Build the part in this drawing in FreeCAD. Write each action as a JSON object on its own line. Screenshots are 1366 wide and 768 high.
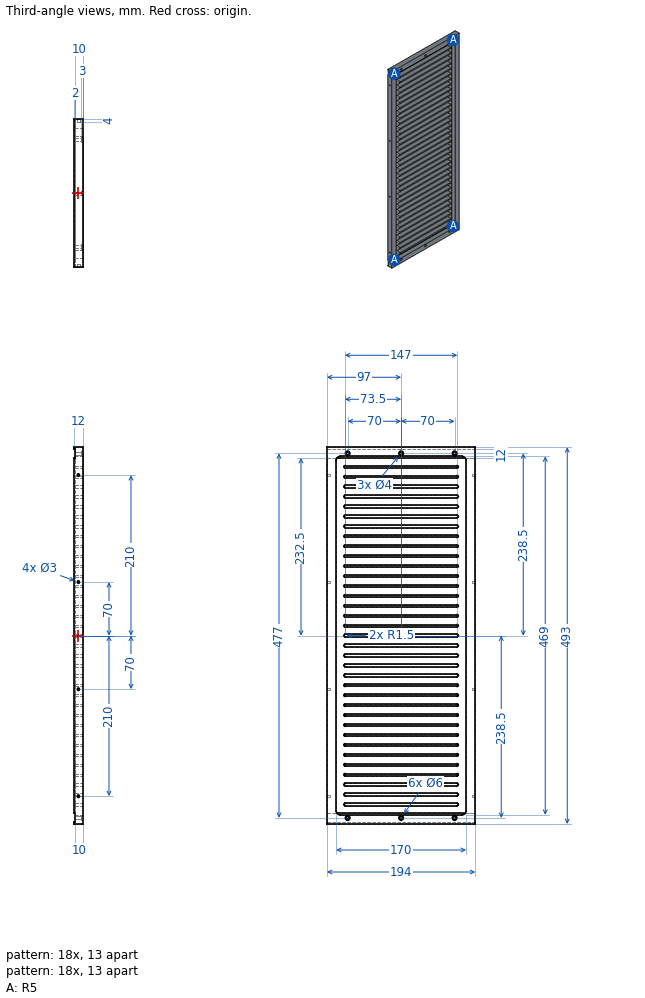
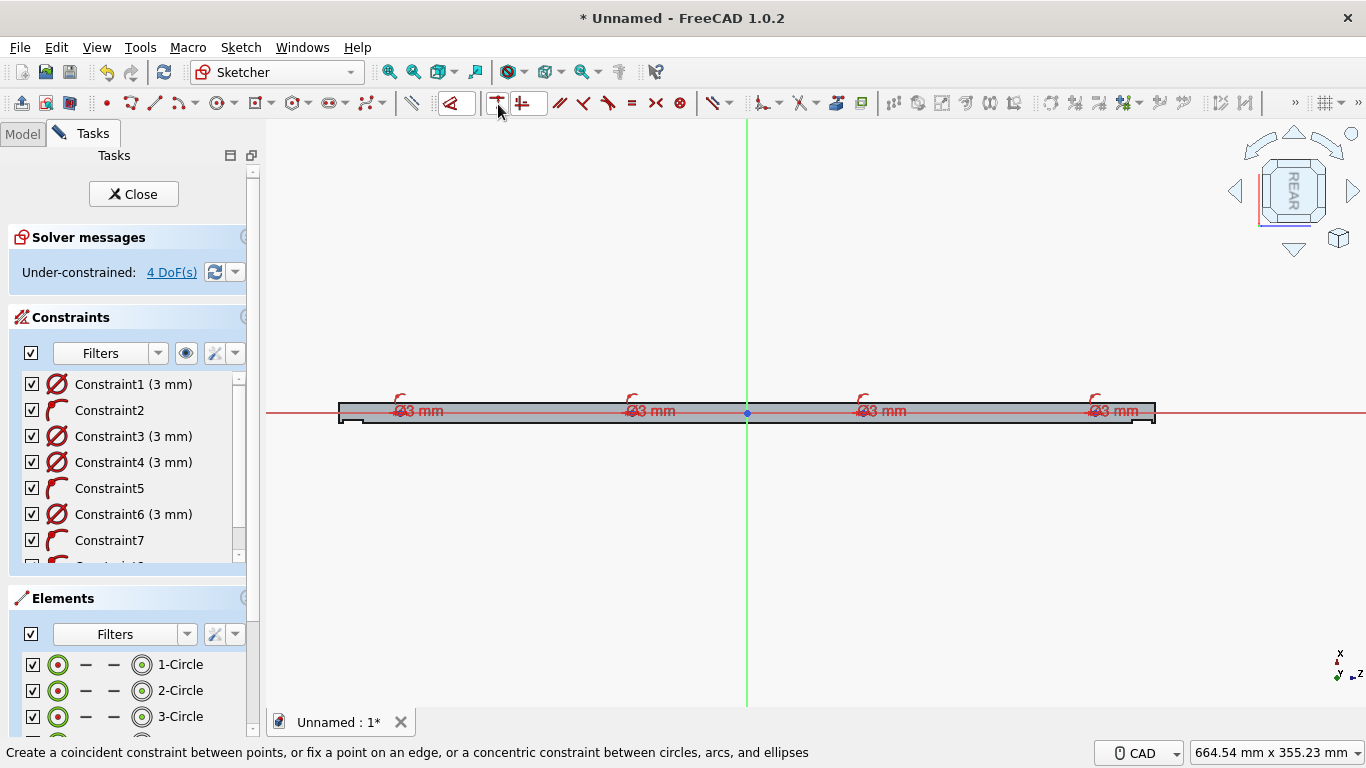
{"action": "left_click", "coordinate": [863, 413]}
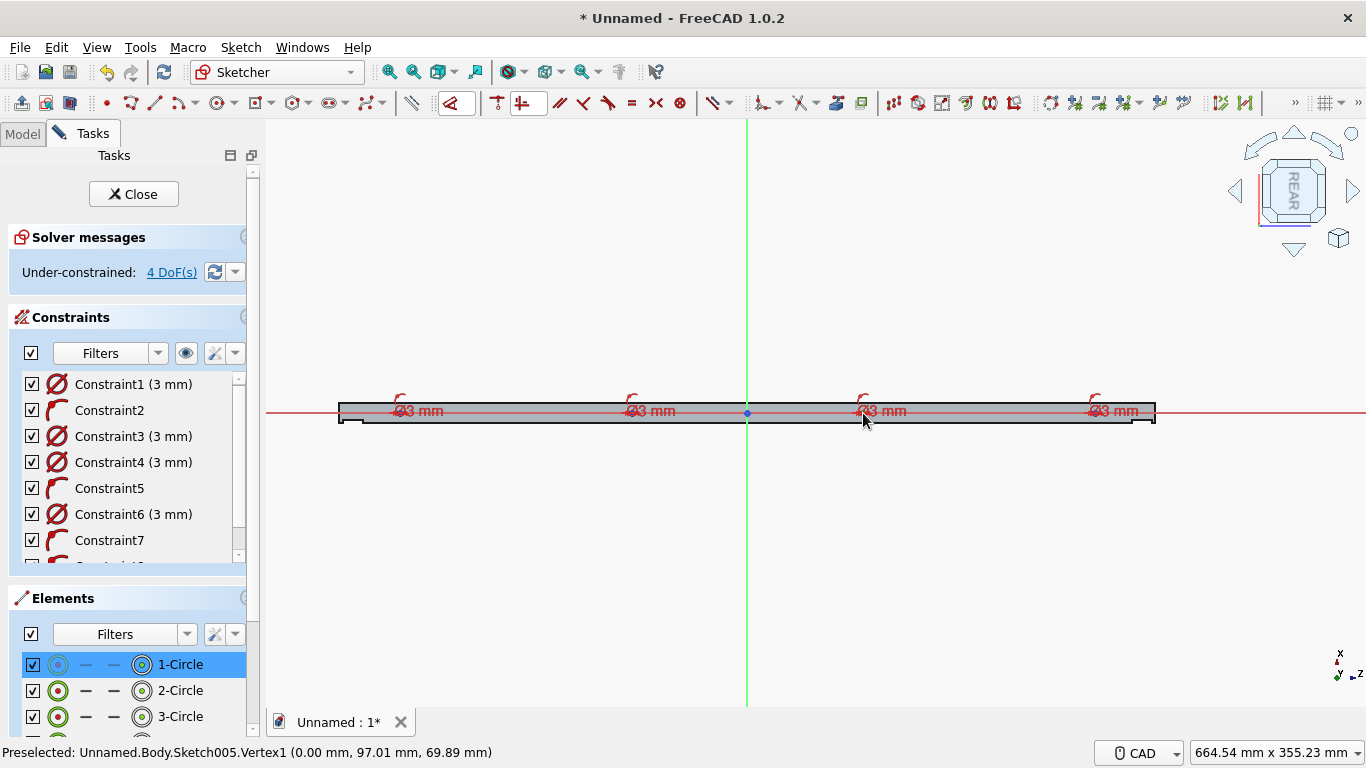
{"action": "key", "text": "l"}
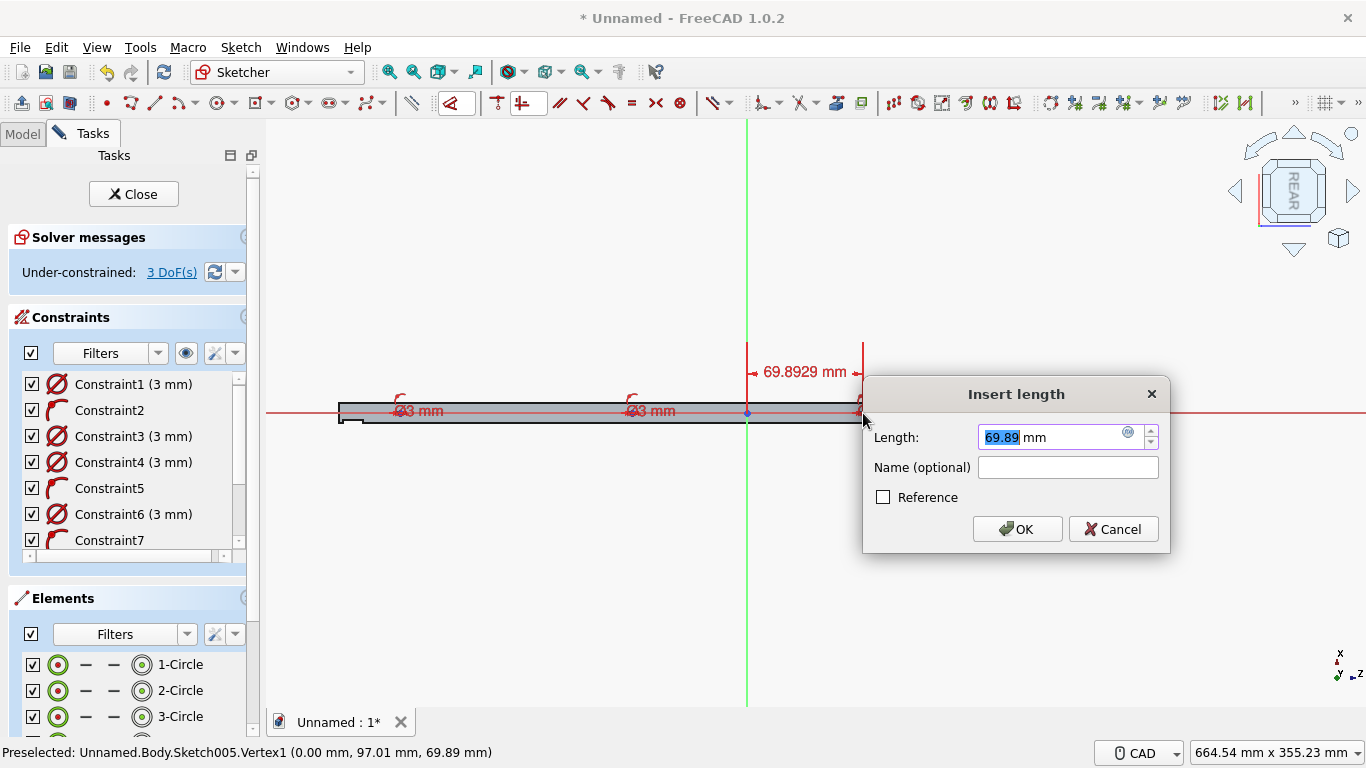
{"action": "type", "text": "70"}
{"action": "key", "text": "Return"}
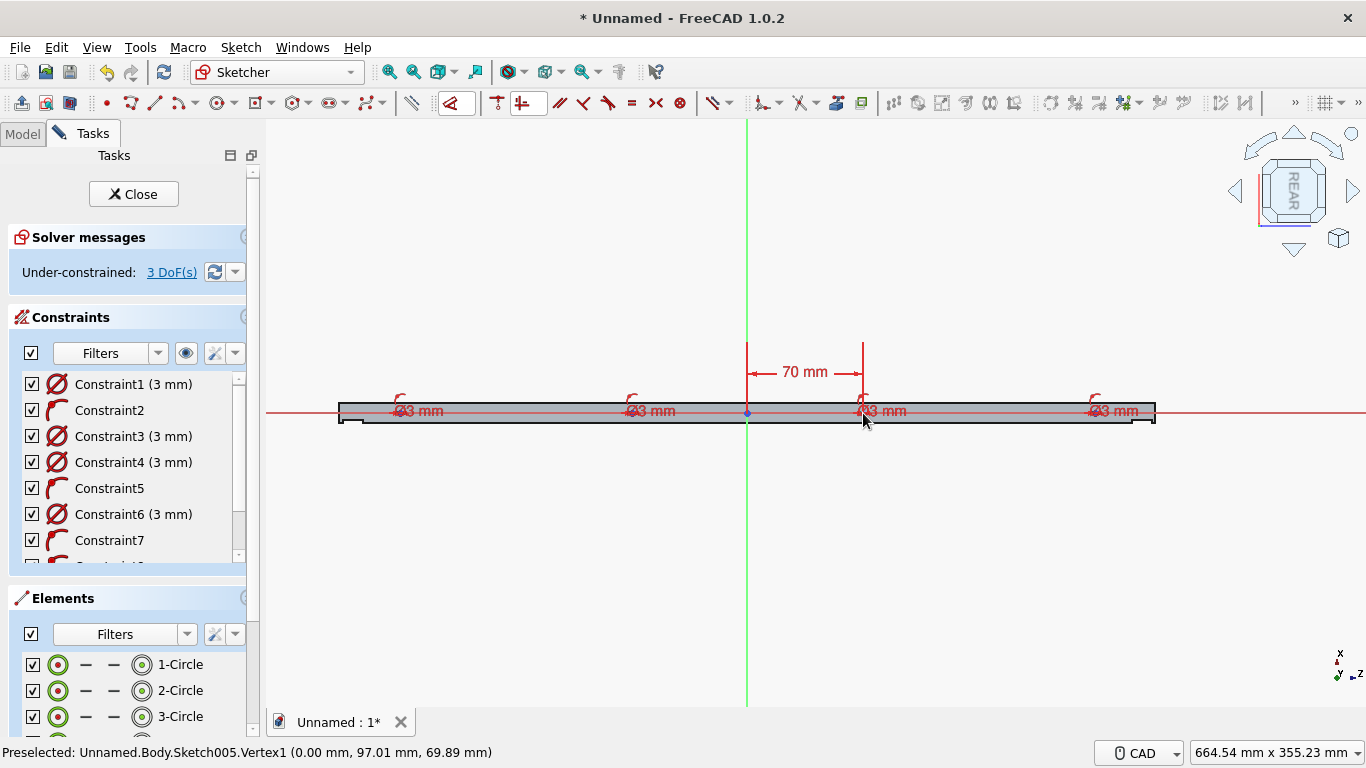
{"action": "left_click", "coordinate": [632, 413]}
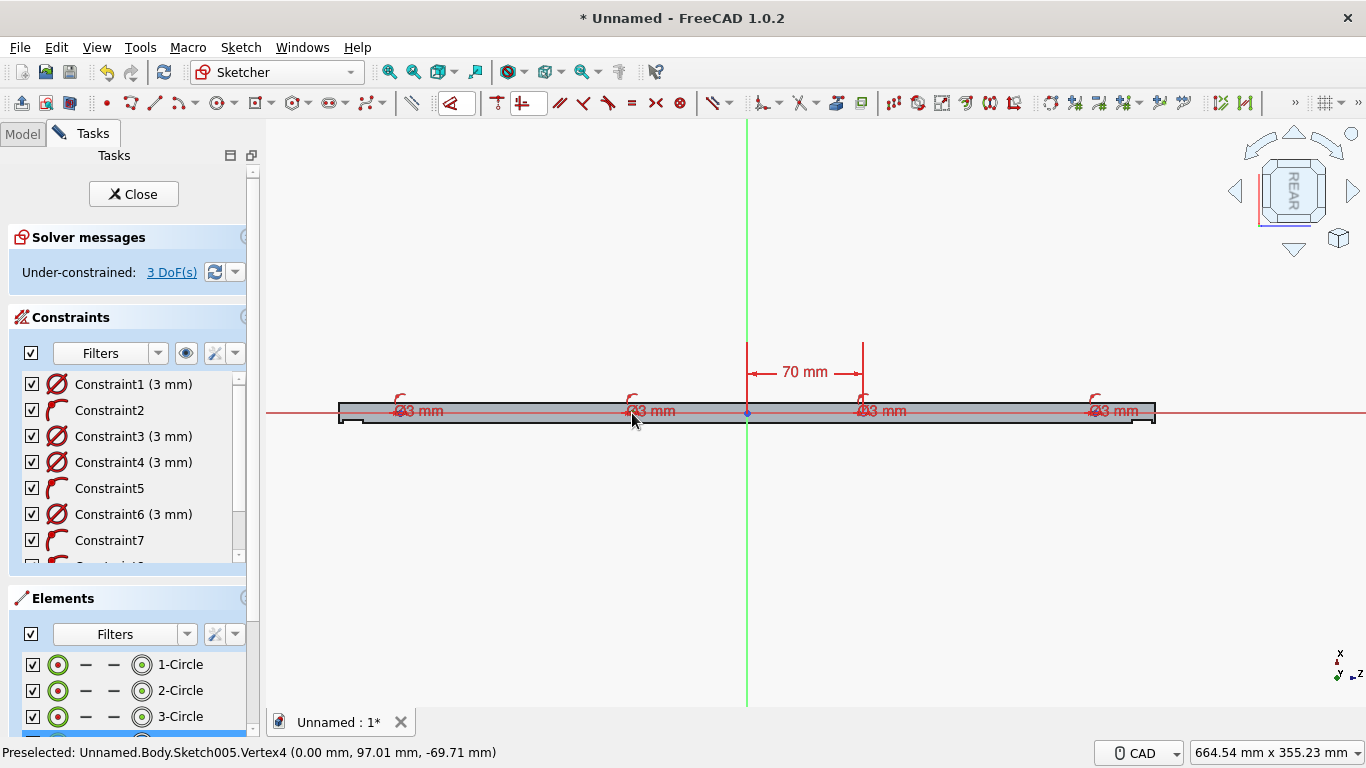
{"action": "left_click", "coordinate": [470, 104]}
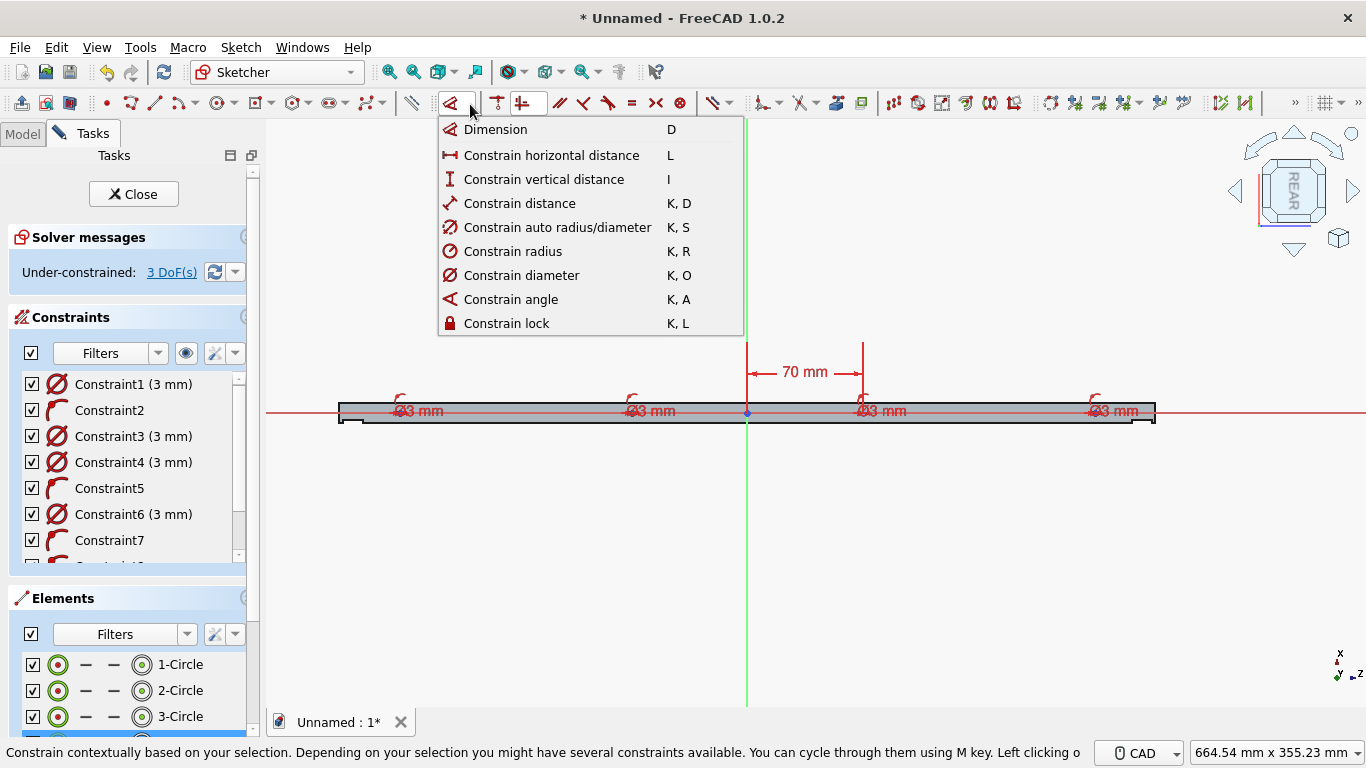
{"action": "left_click", "coordinate": [591, 155]}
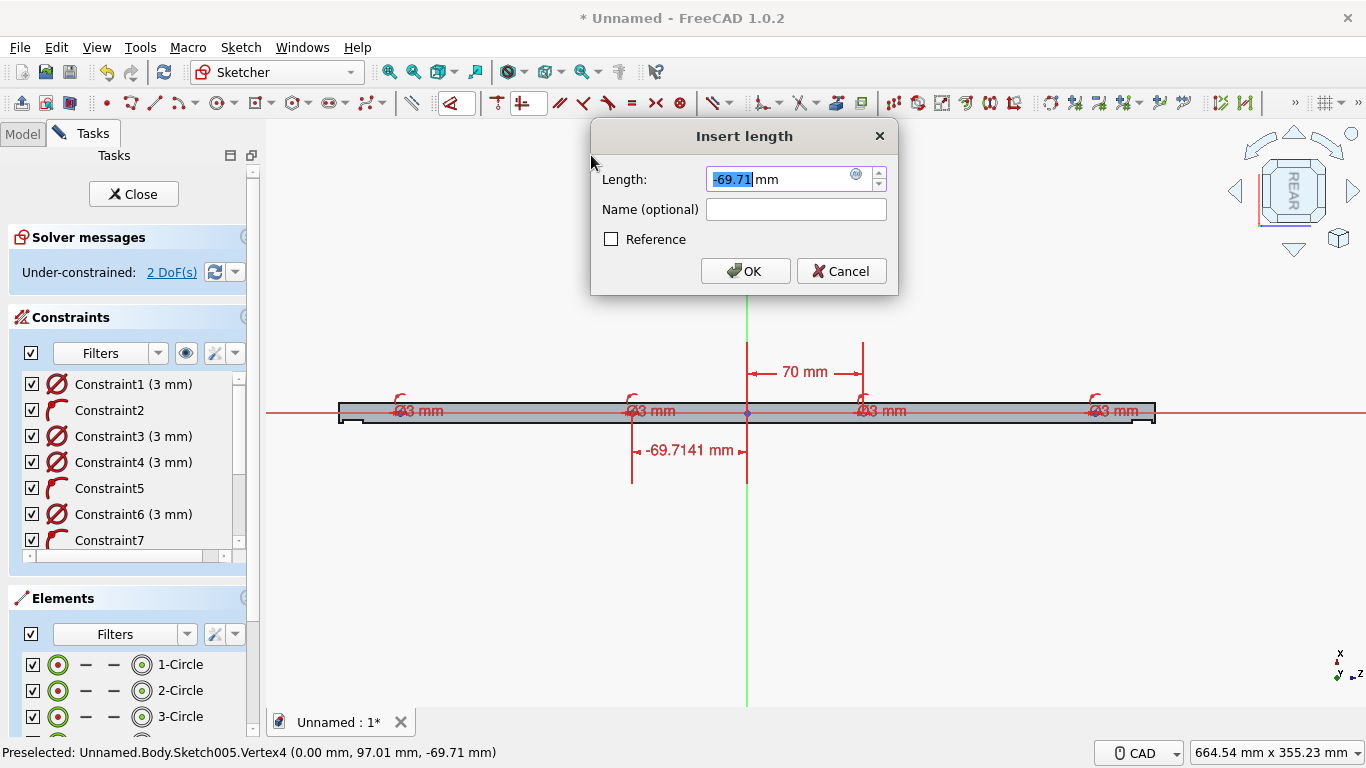
{"action": "type", "text": "-70"}
{"action": "key", "text": "Return"}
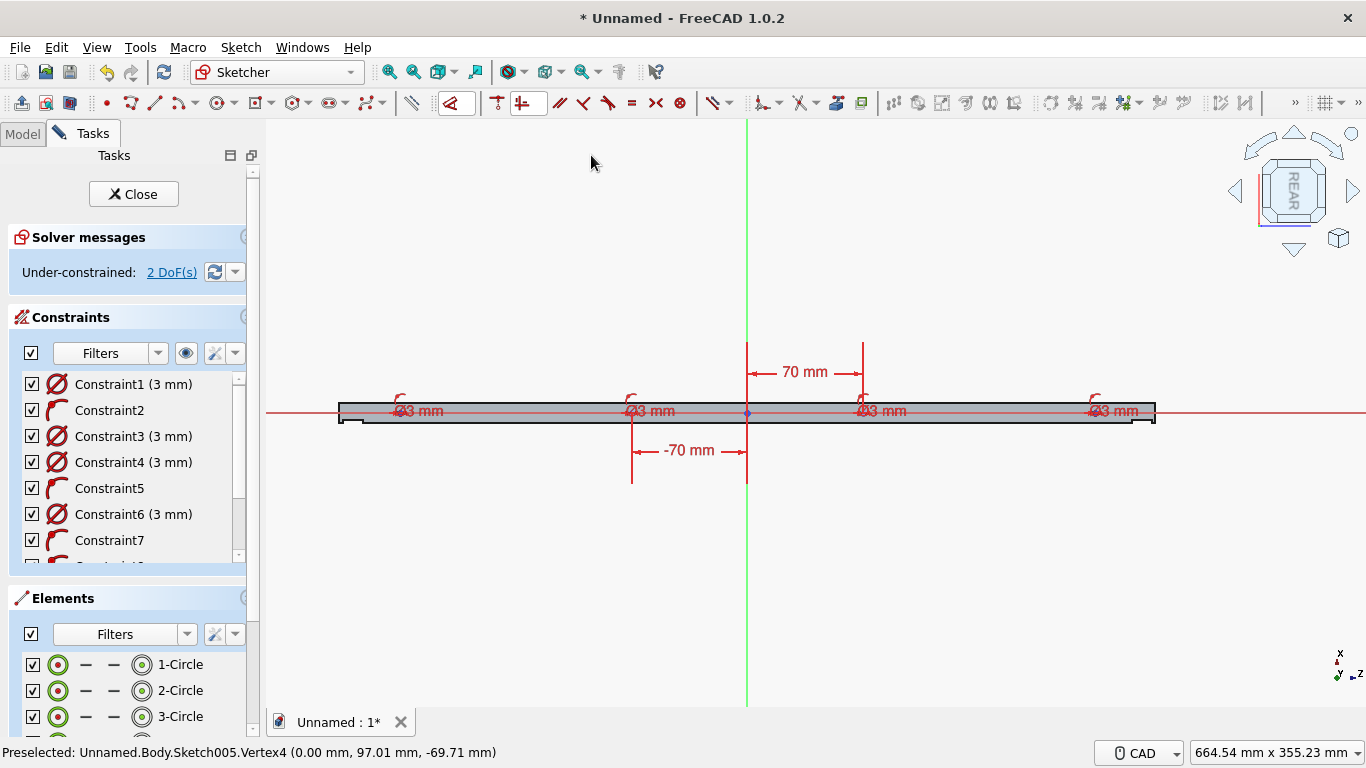
{"action": "left_click", "coordinate": [1095, 413]}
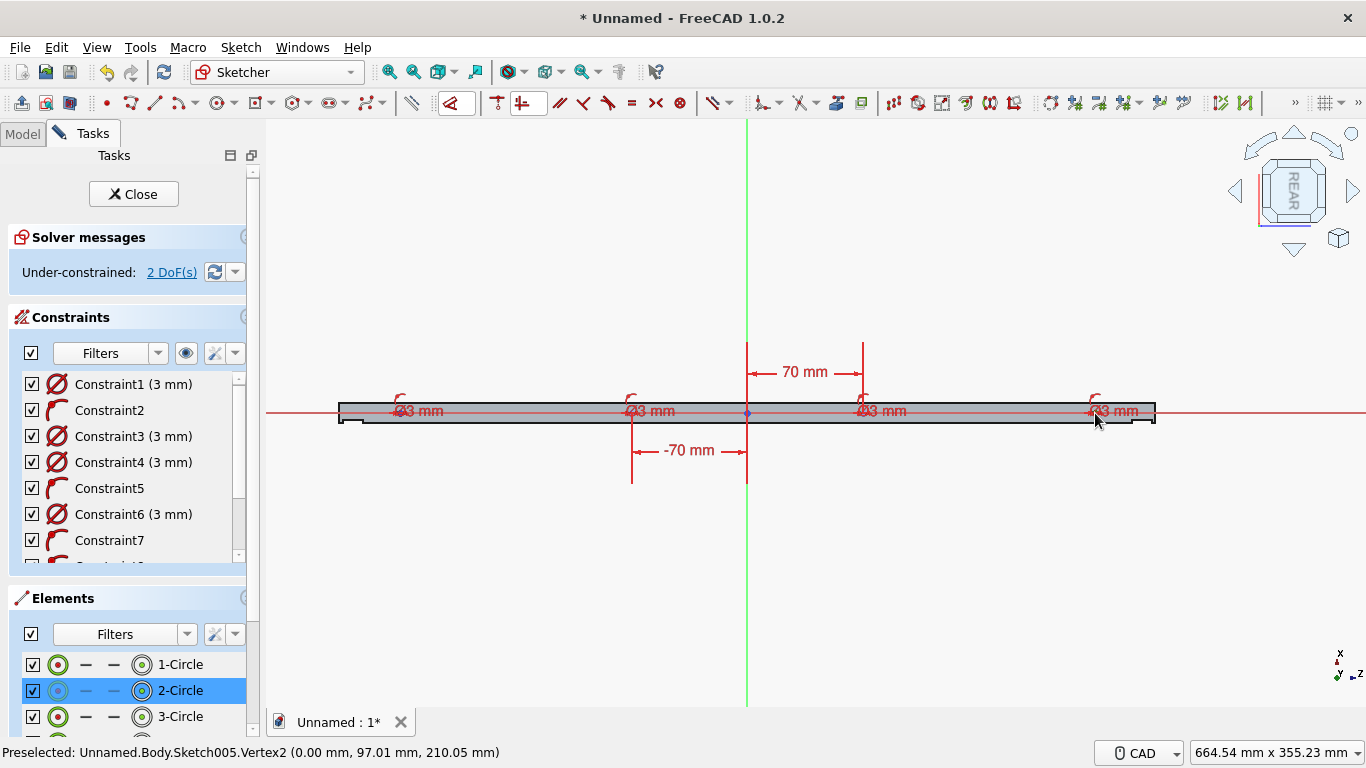
{"action": "key", "text": "l"}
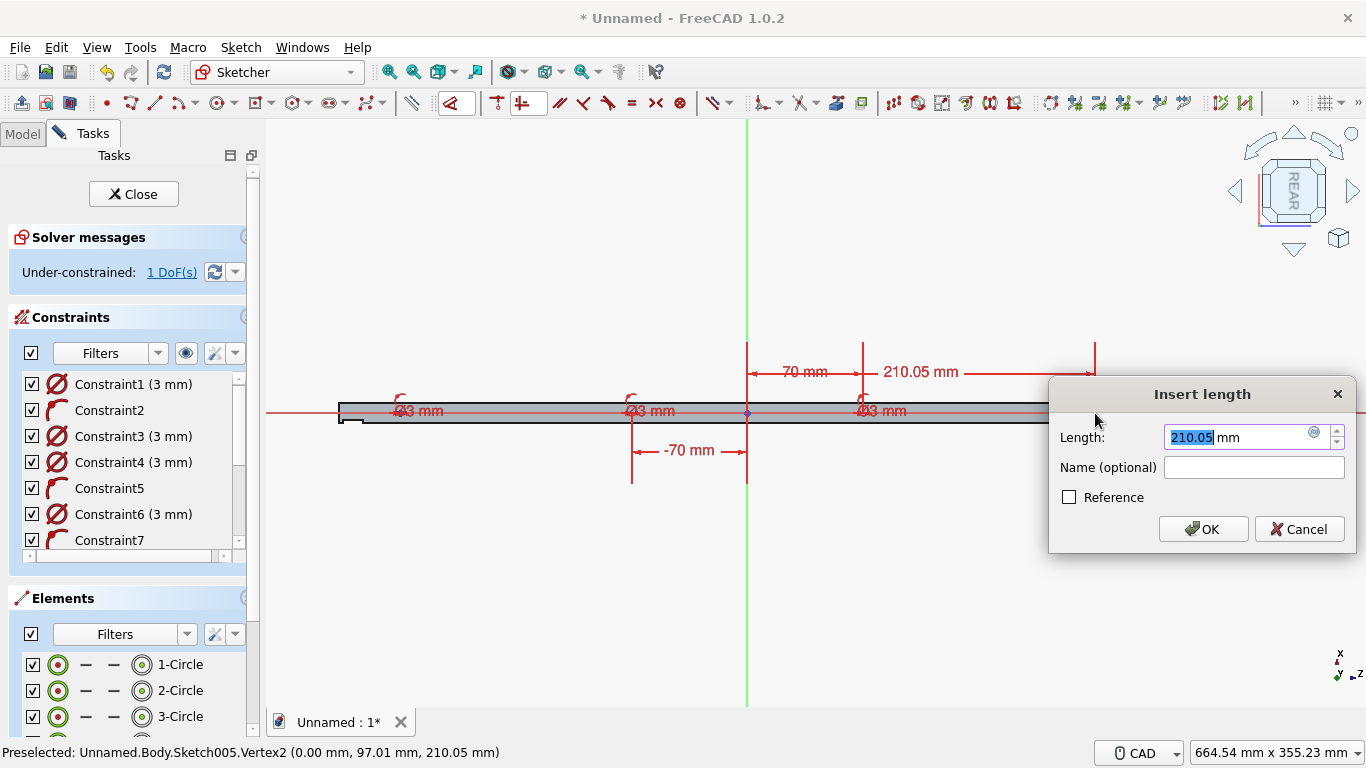
{"action": "type", "text": "210"}
{"action": "key", "text": "Return"}